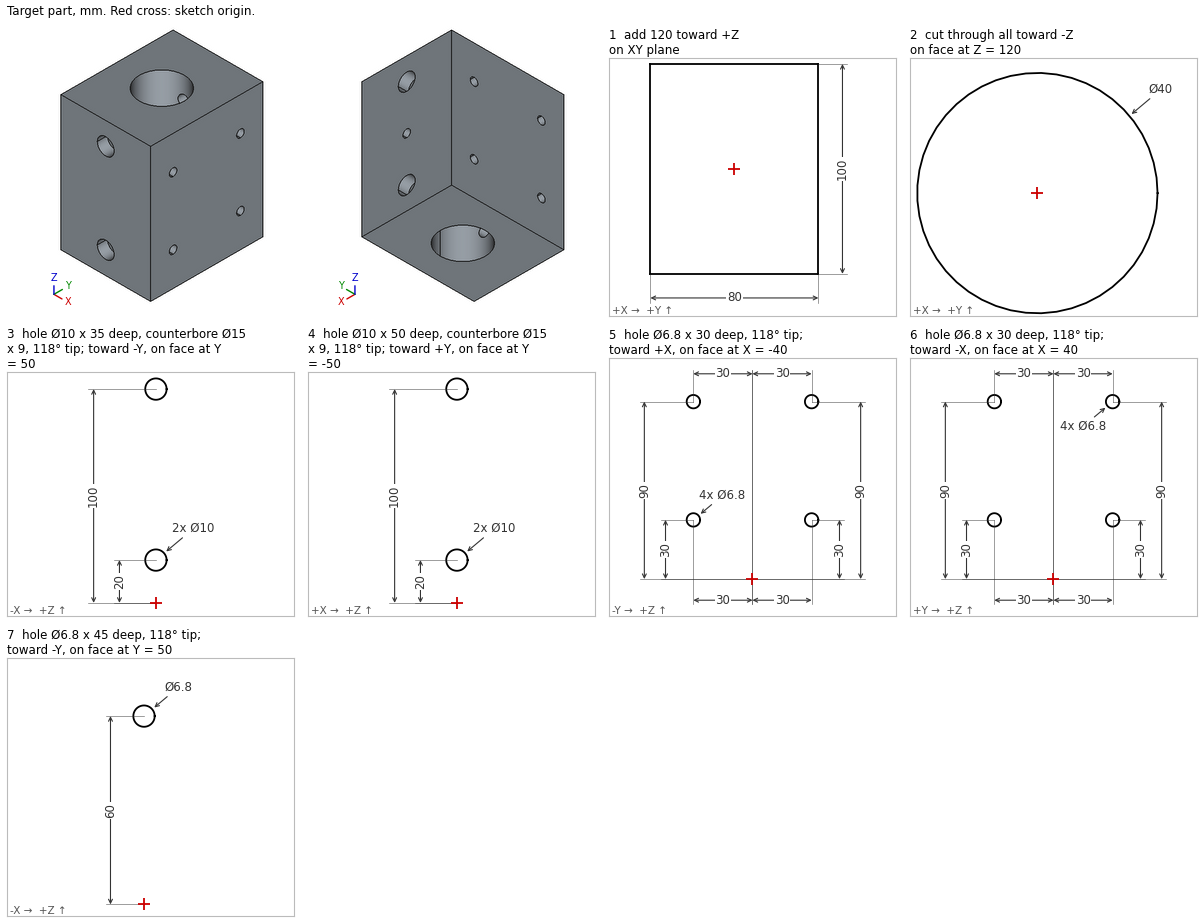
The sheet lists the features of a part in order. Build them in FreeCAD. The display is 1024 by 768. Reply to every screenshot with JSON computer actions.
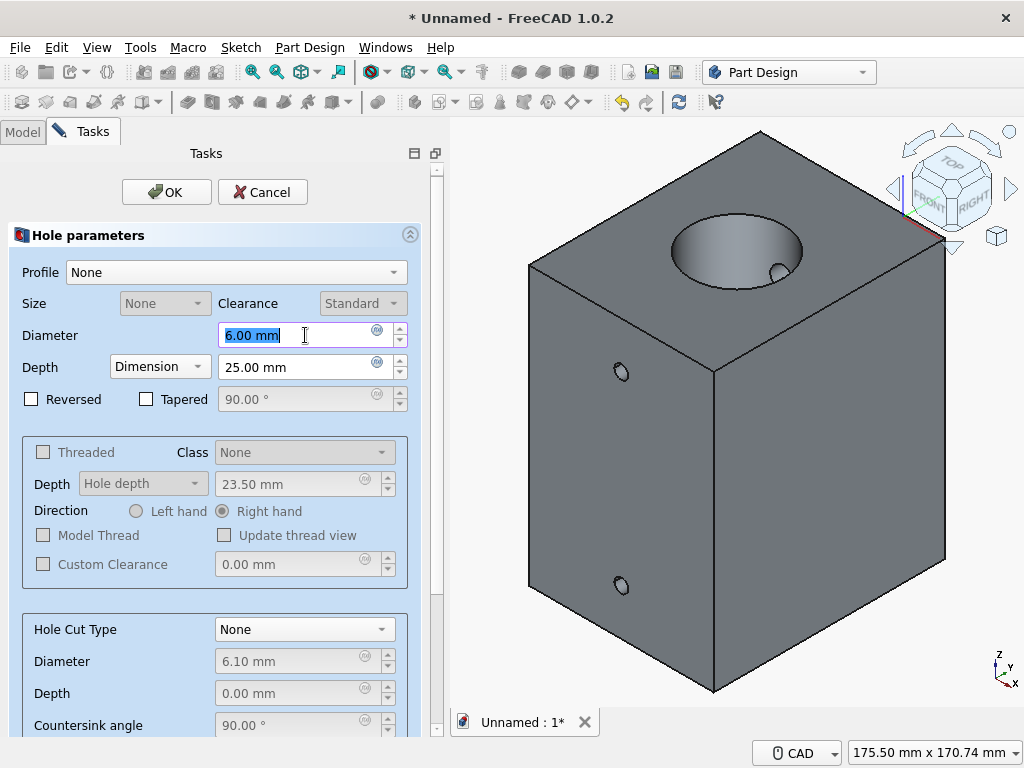
{"action": "type", "text": "10"}
{"action": "key", "text": "Tab"}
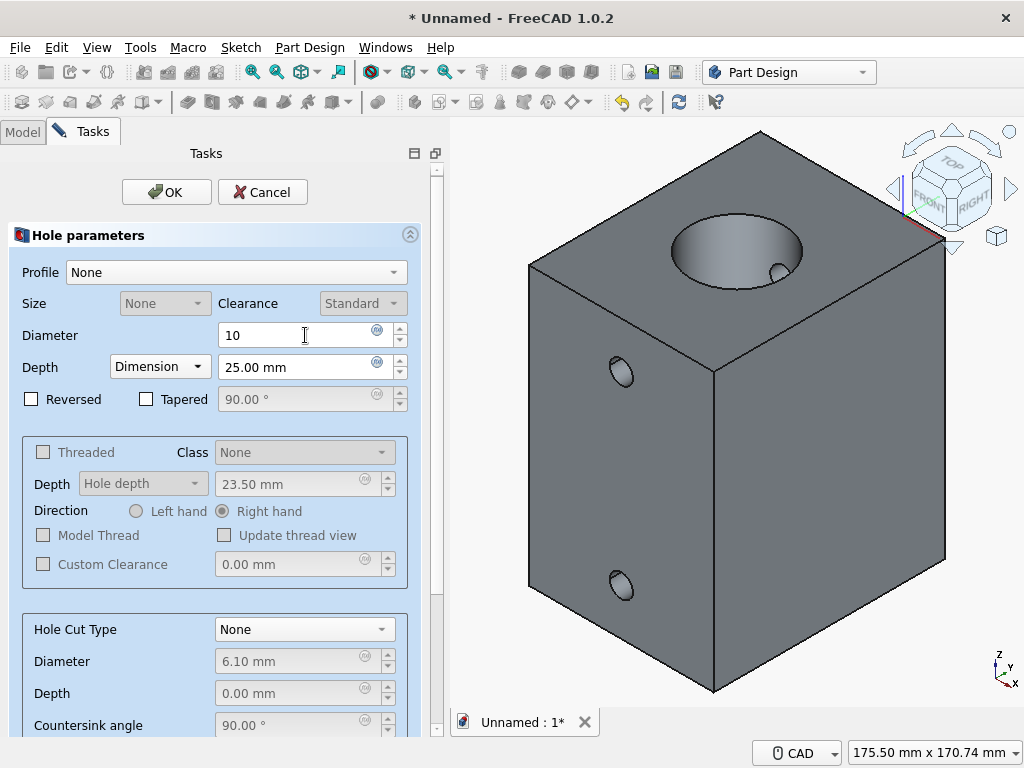
{"action": "triple_click", "coordinate": [305, 367]}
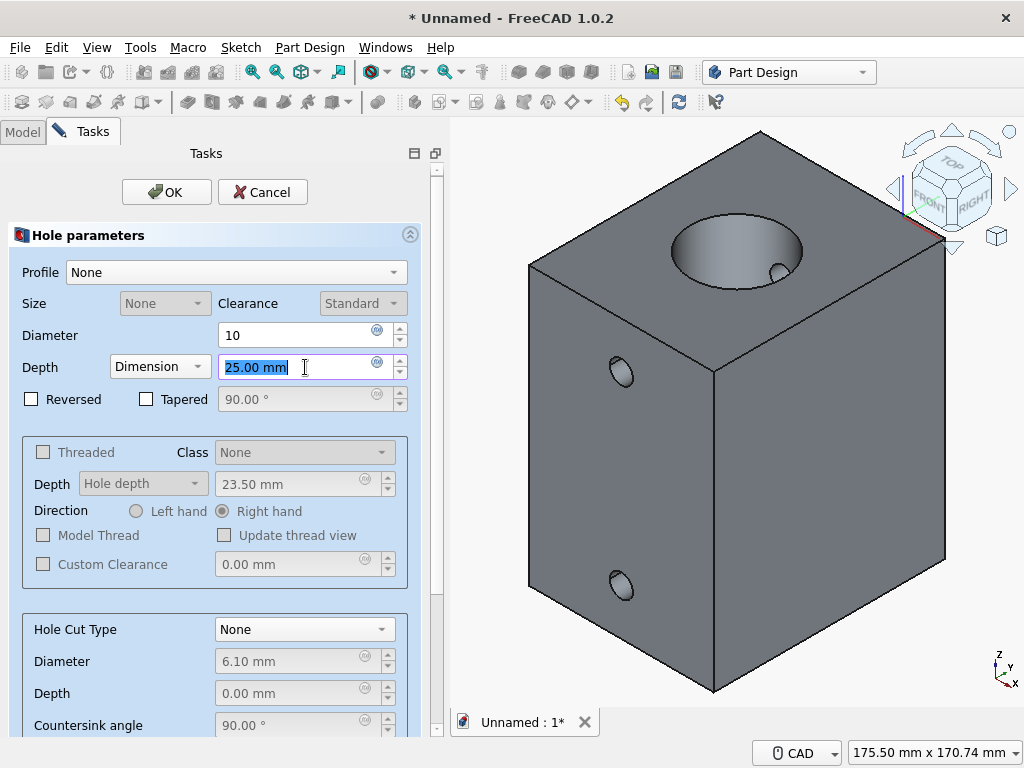
{"action": "type", "text": "50"}
{"action": "key", "text": "Tab"}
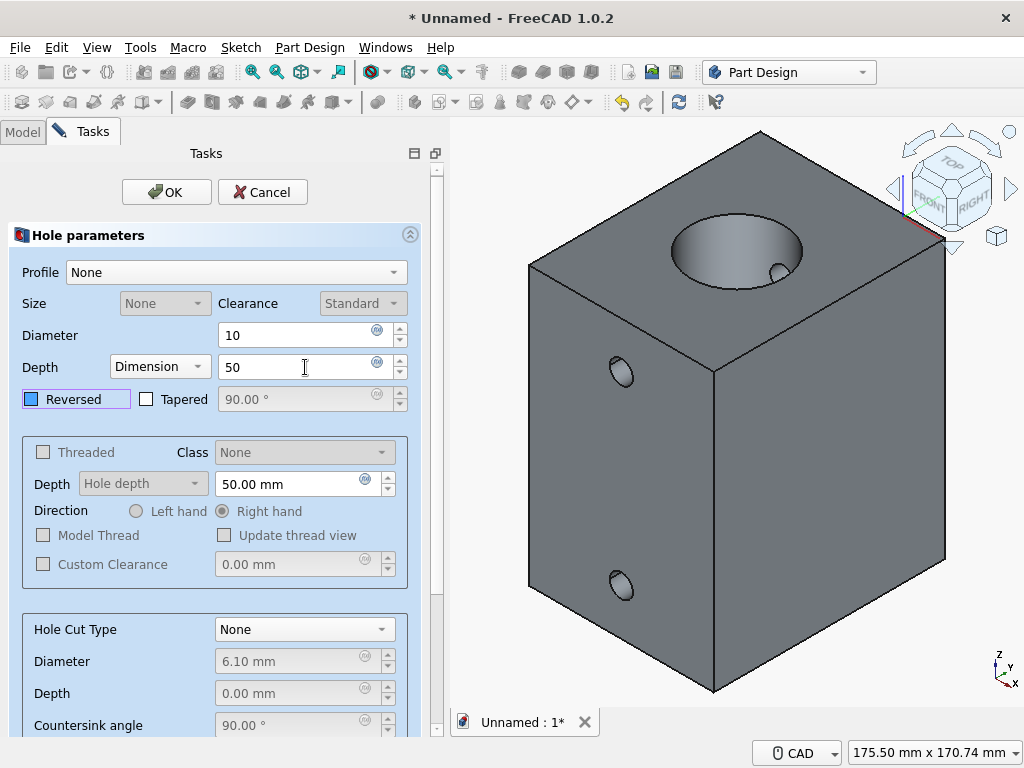
{"action": "left_click", "coordinate": [306, 630]}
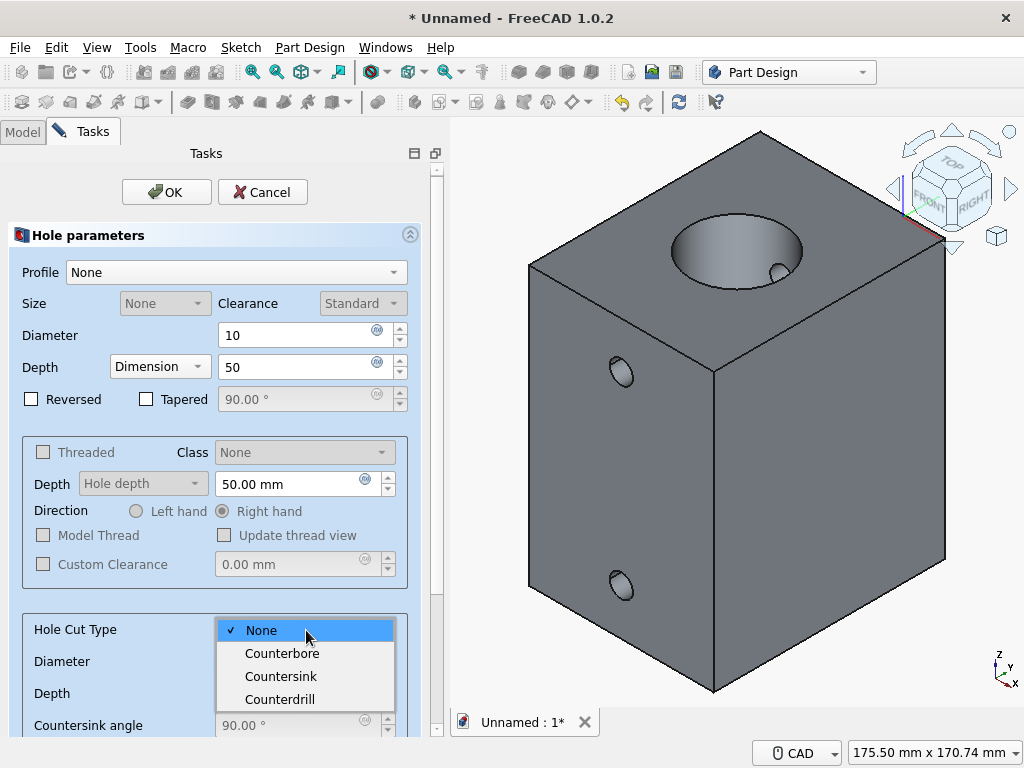
{"action": "left_click", "coordinate": [304, 654]}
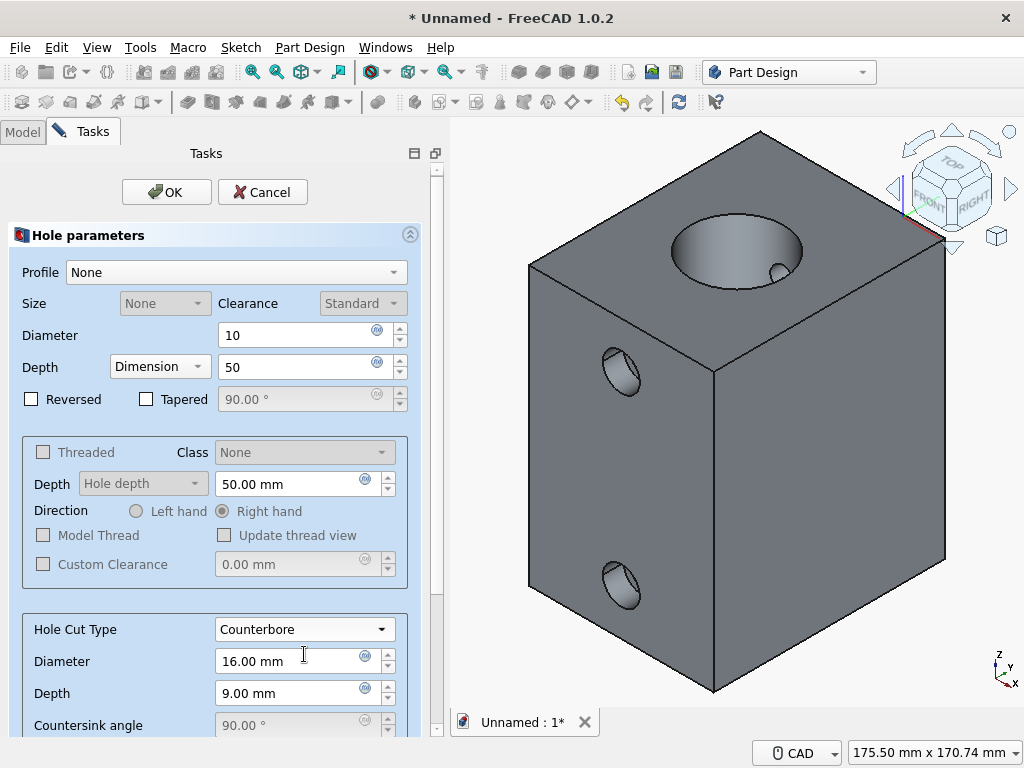
{"action": "triple_click", "coordinate": [298, 661]}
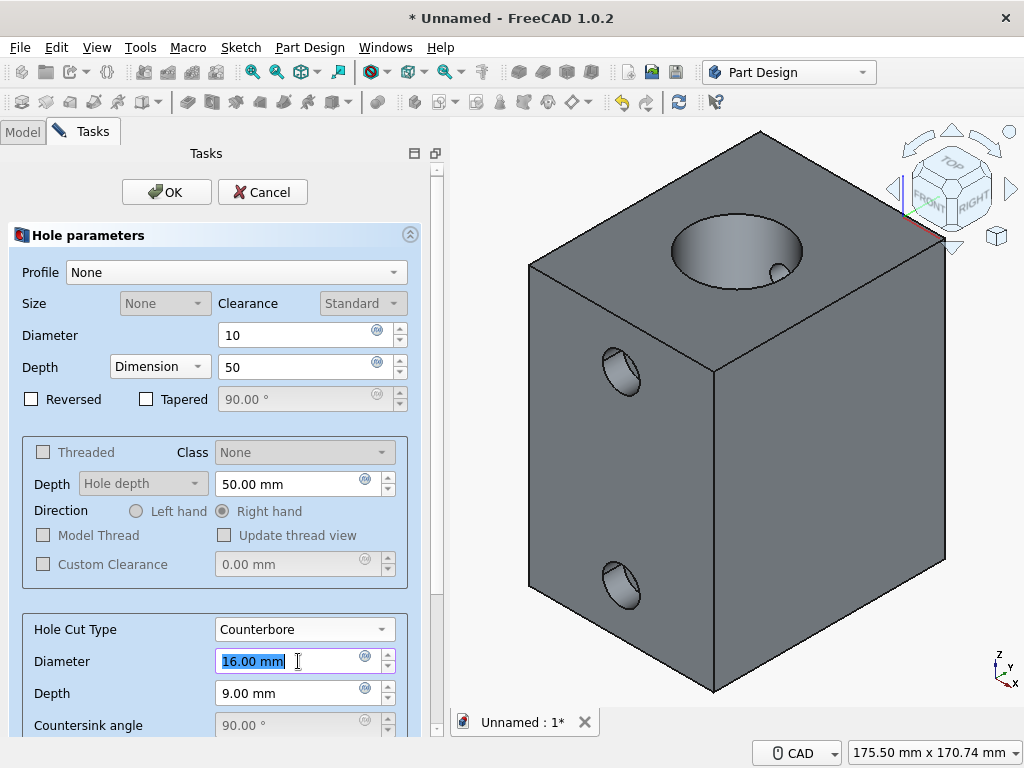
{"action": "type", "text": "15"}
{"action": "key", "text": "Tab"}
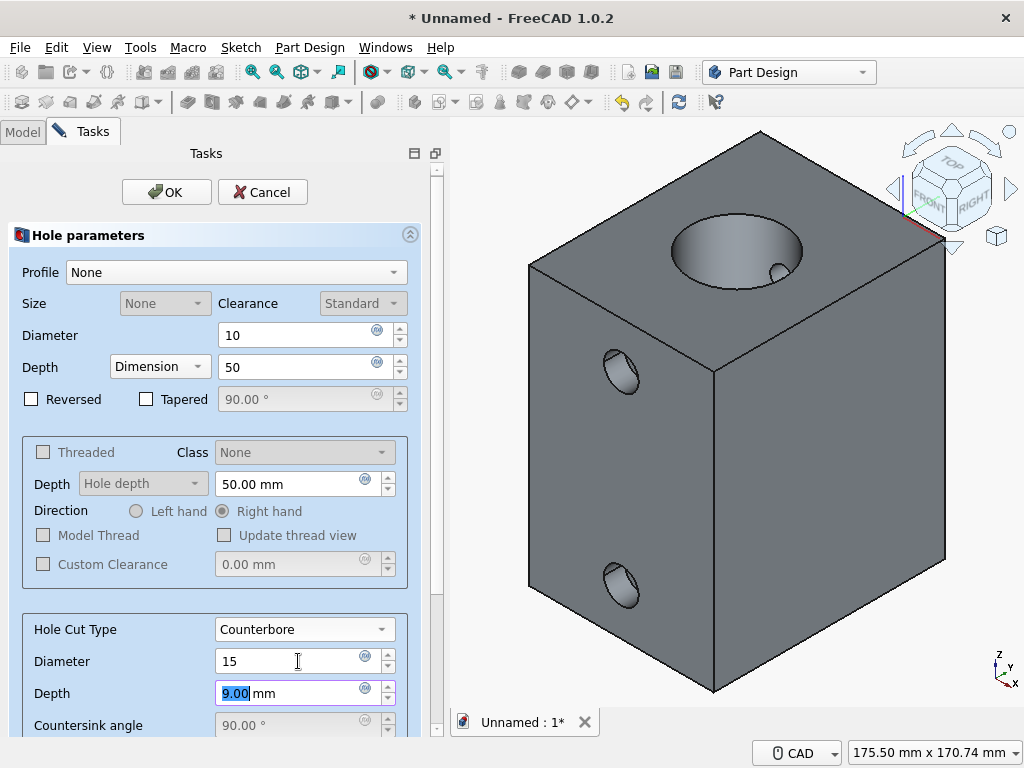
{"action": "type", "text": "9"}
{"action": "key", "text": "Tab"}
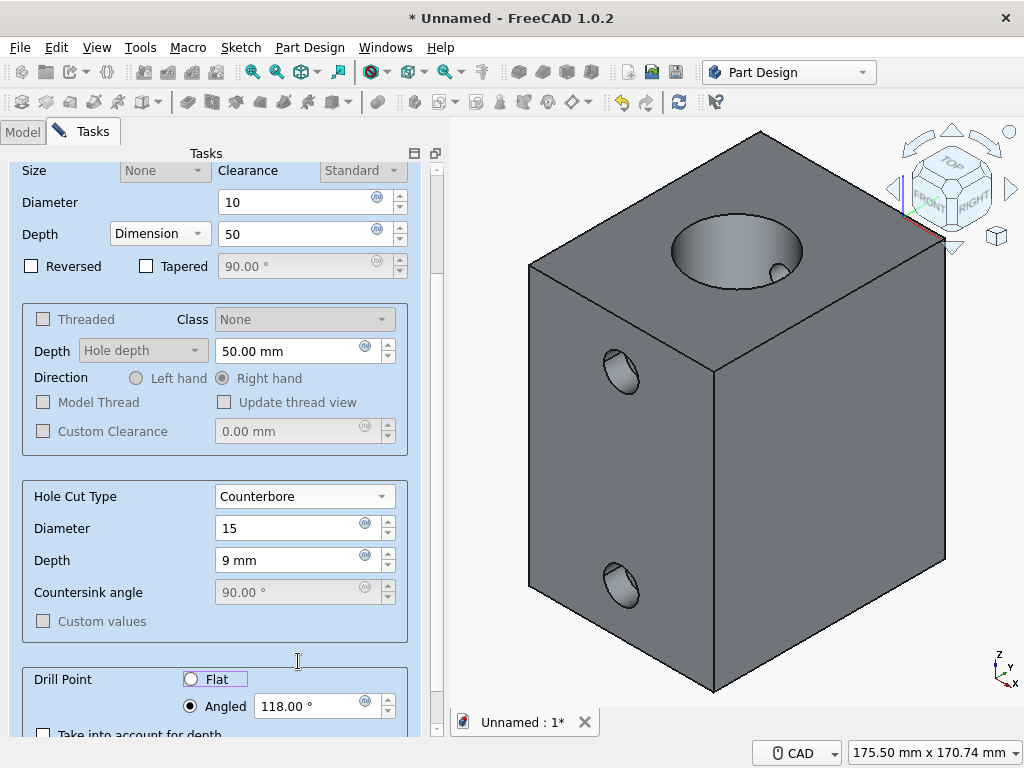
{"action": "scroll", "coordinate": [437, 450], "scroll_direction": "up", "scroll_amount": 3}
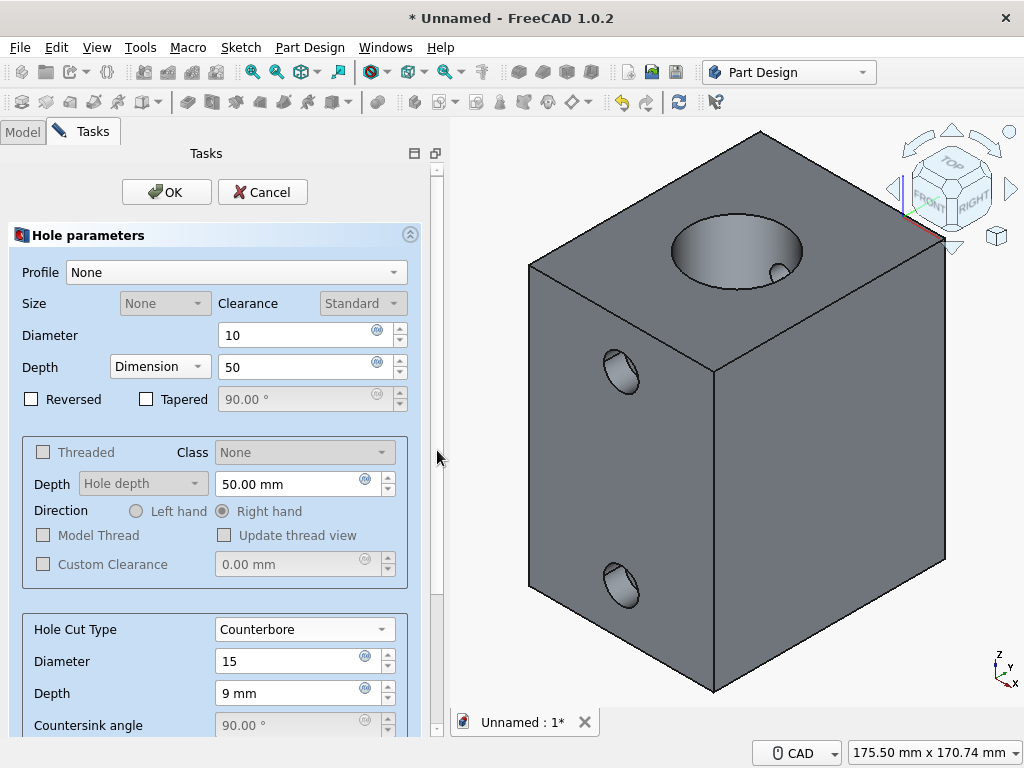
{"action": "left_click", "coordinate": [167, 192]}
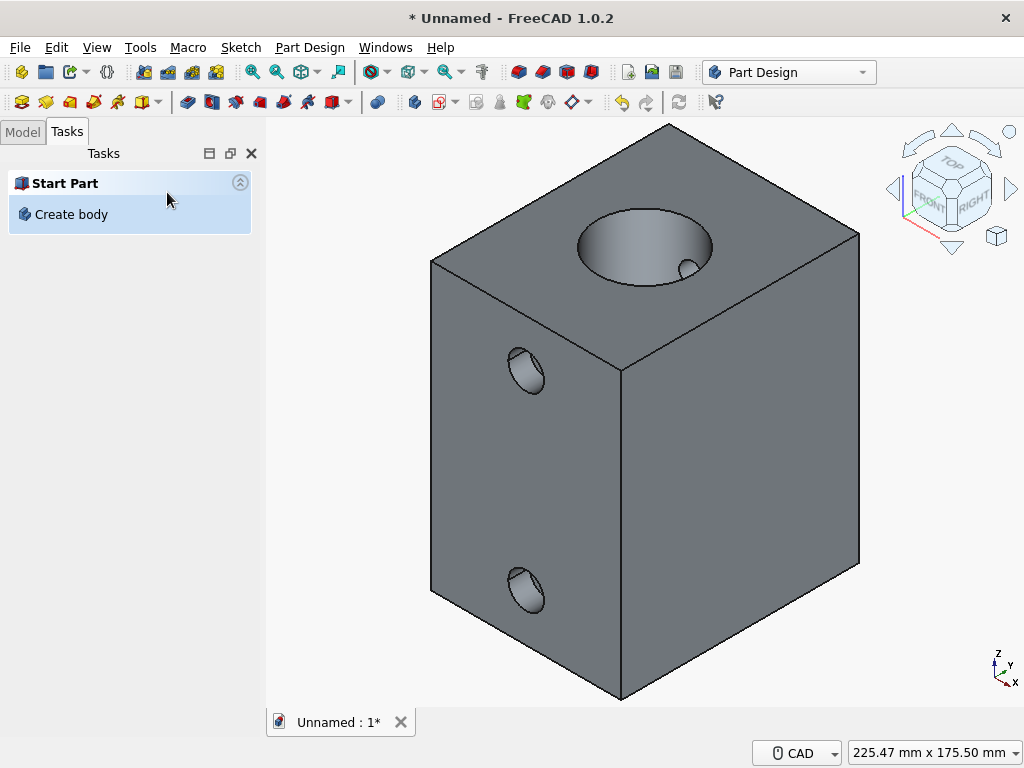
{"action": "key", "text": "6"}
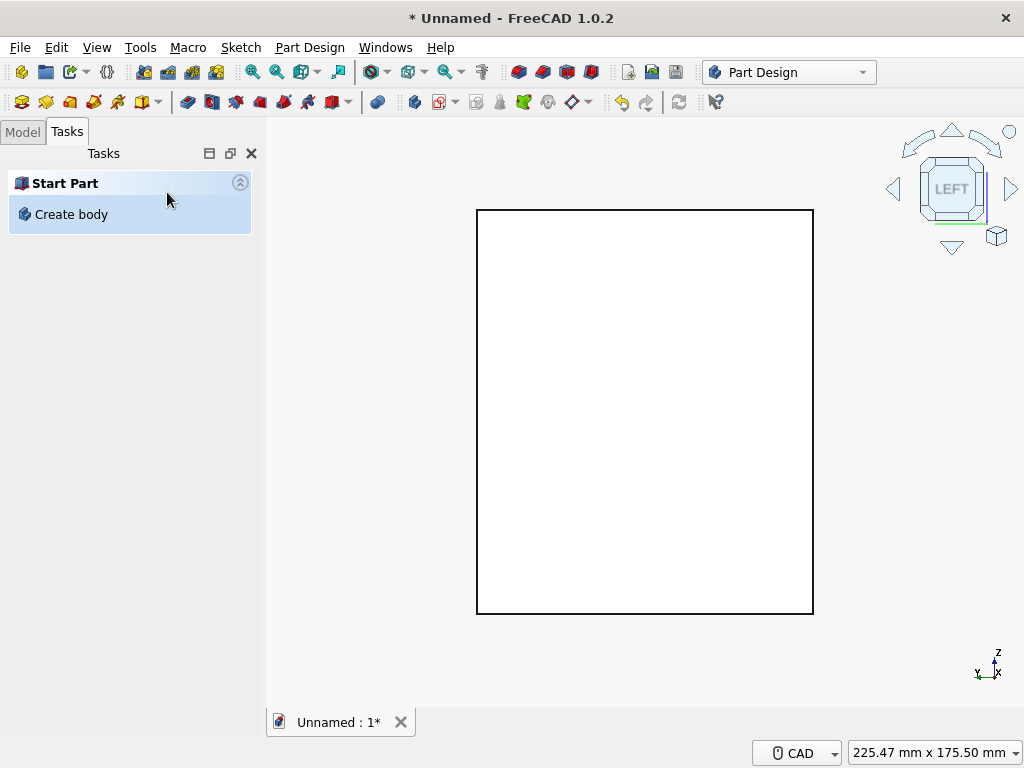
{"action": "left_click", "coordinate": [645, 411]}